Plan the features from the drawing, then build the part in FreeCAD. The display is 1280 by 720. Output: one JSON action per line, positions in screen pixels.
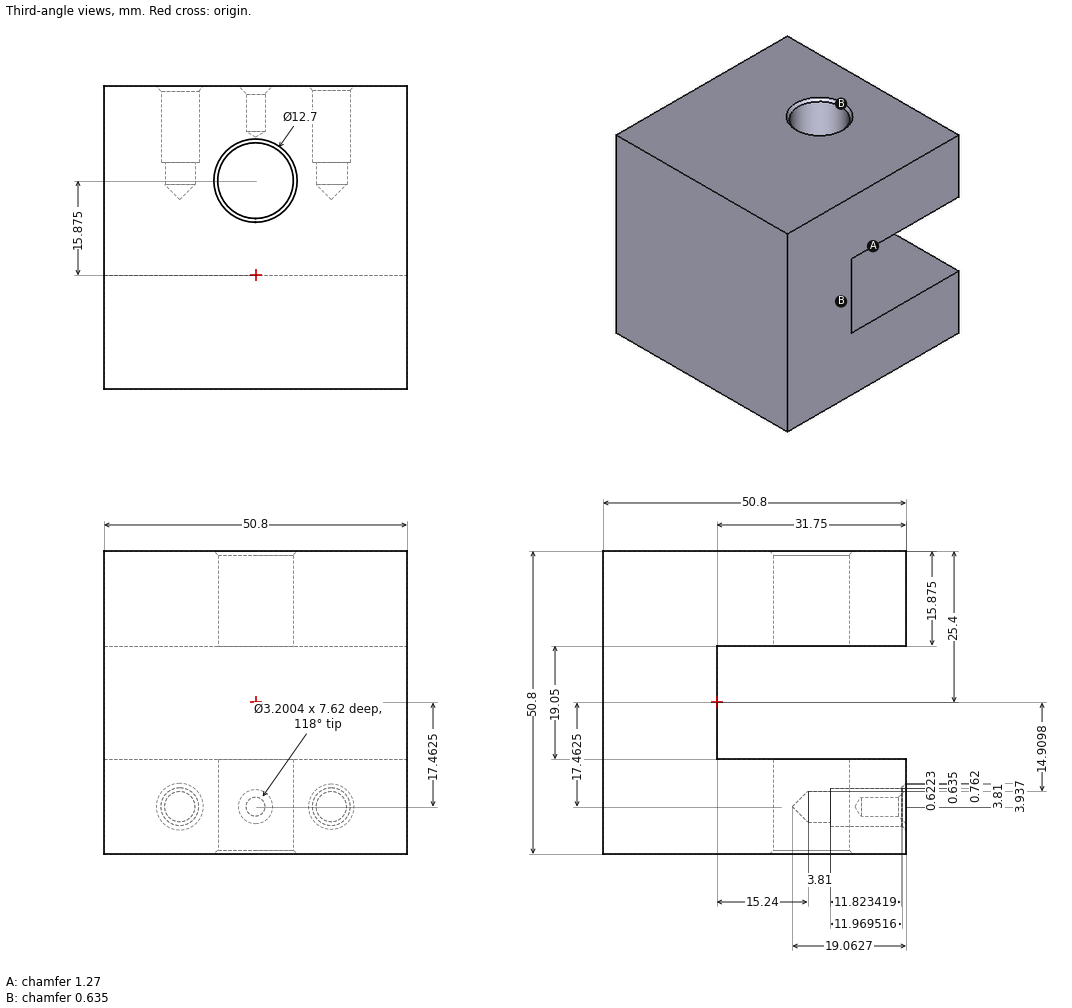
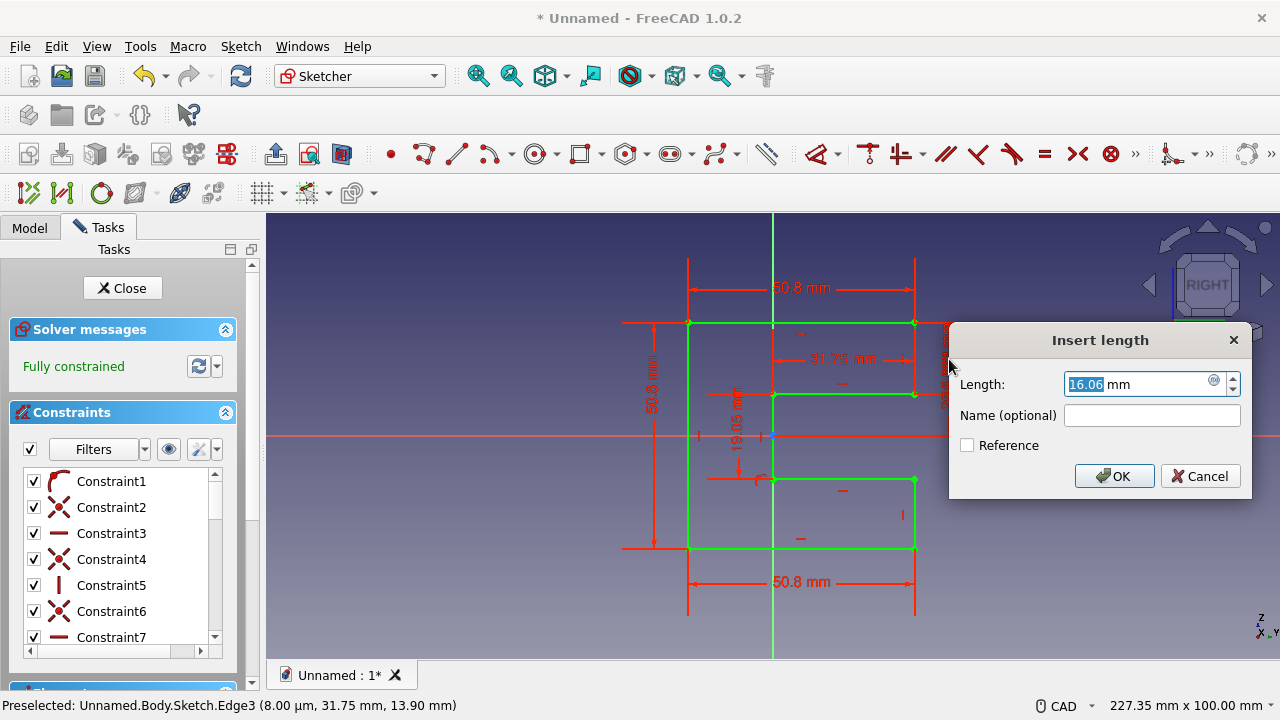
{"action": "type", "text": "15.875"}
{"action": "key", "text": "Return"}
{"action": "key", "text": "Escape"}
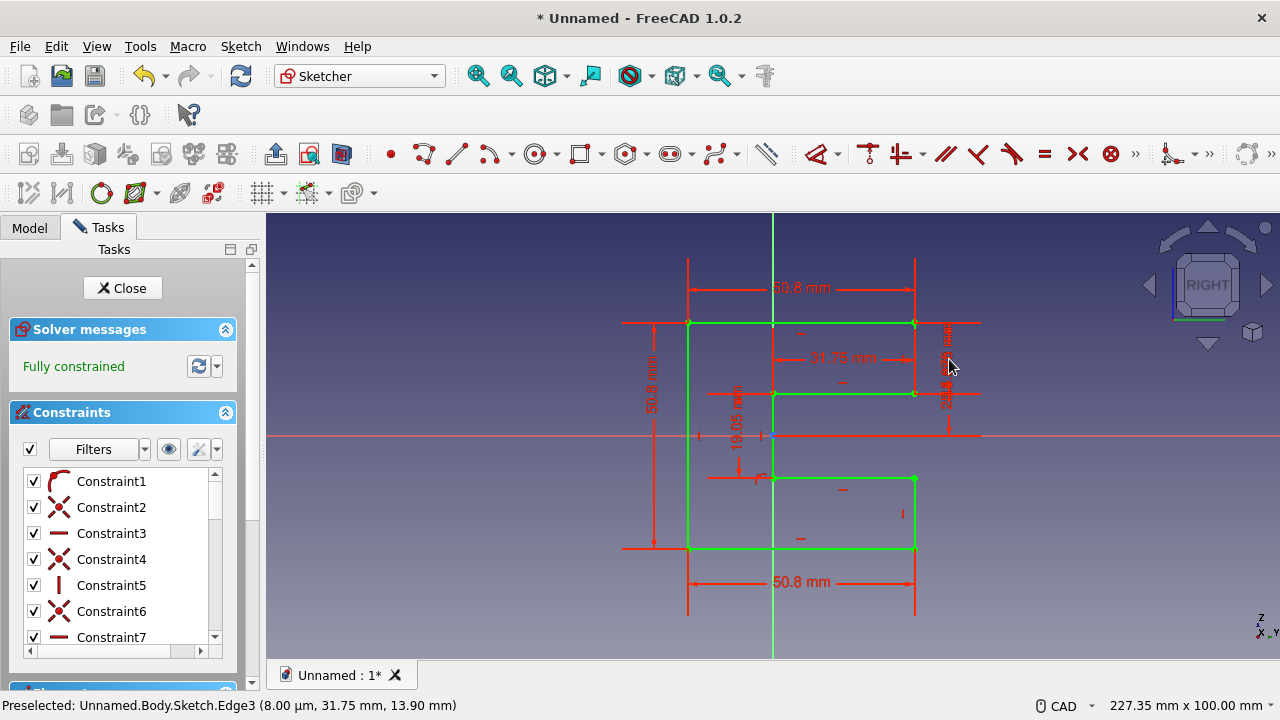
{"action": "left_click", "coordinate": [123, 288]}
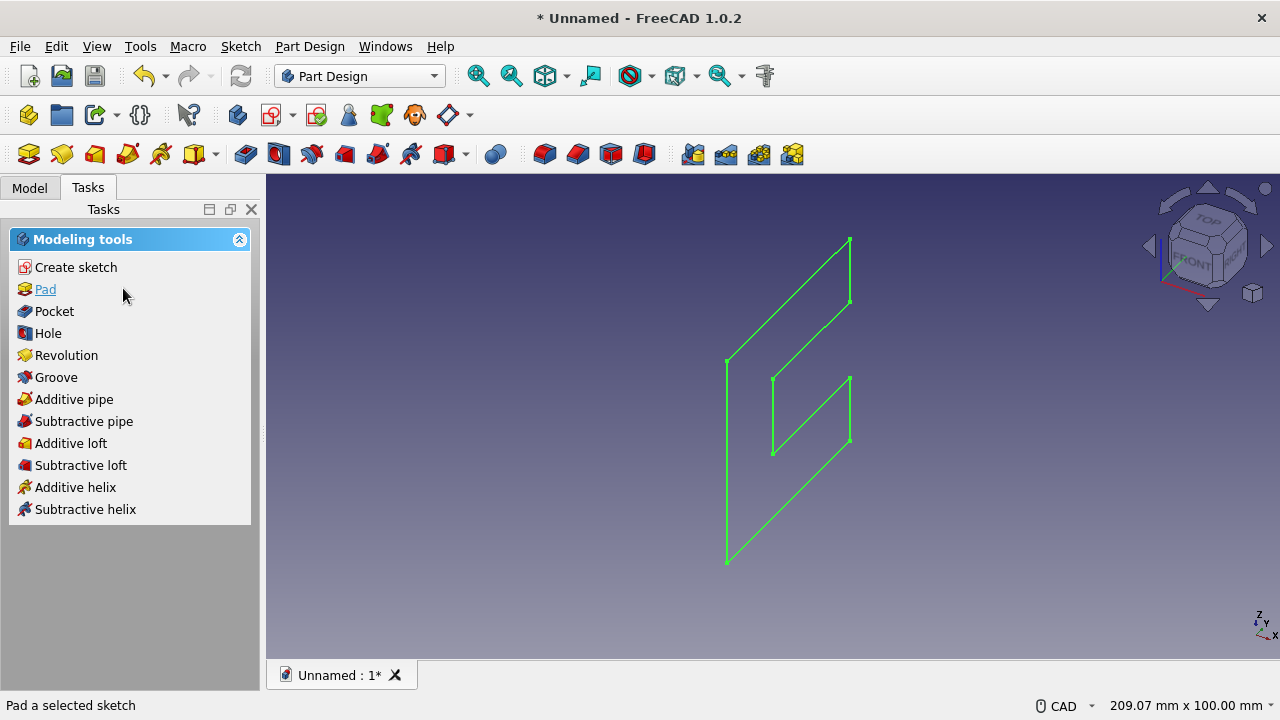
{"action": "left_click", "coordinate": [29, 154]}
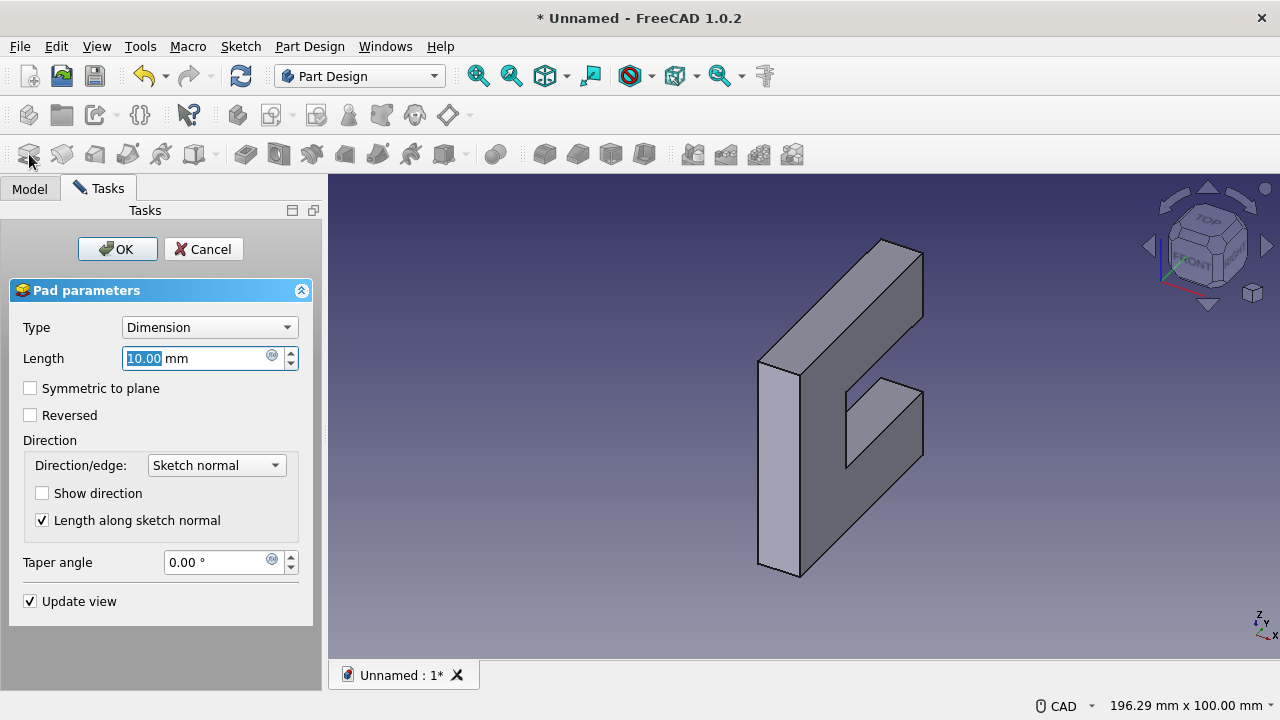
{"action": "type", "text": "50.8"}
{"action": "key", "text": "Tab"}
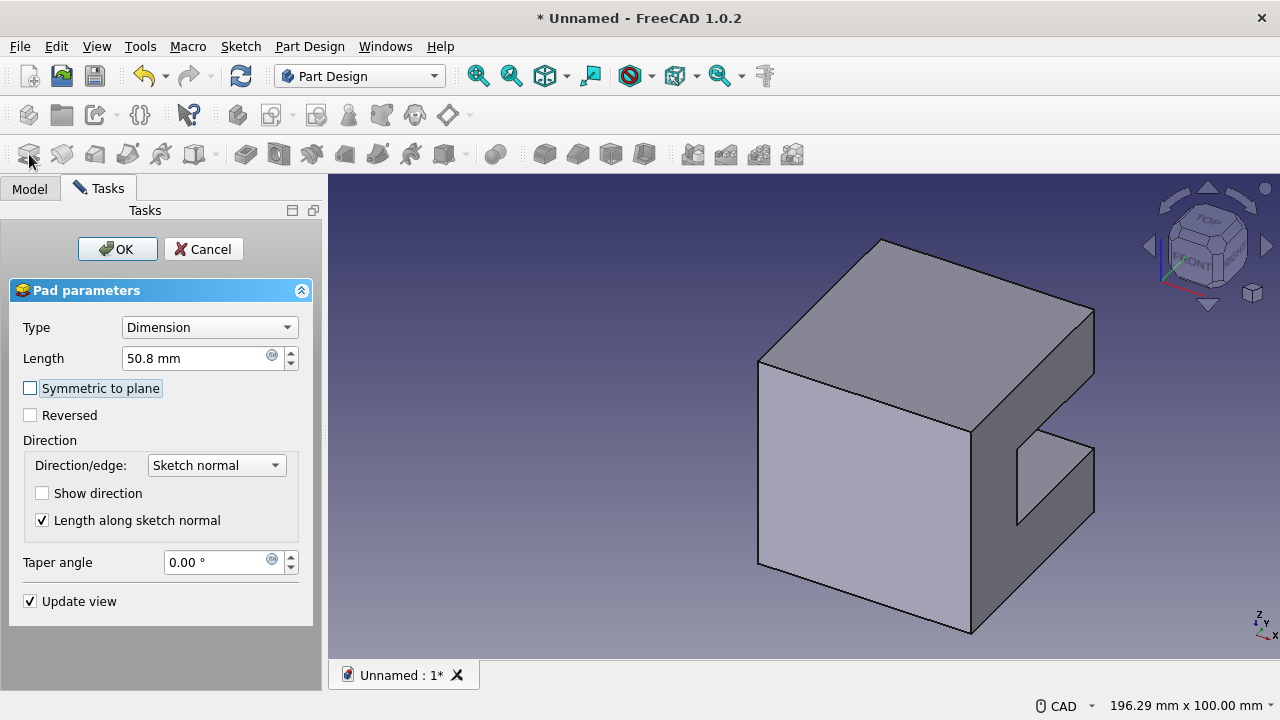
{"action": "left_click", "coordinate": [31, 388]}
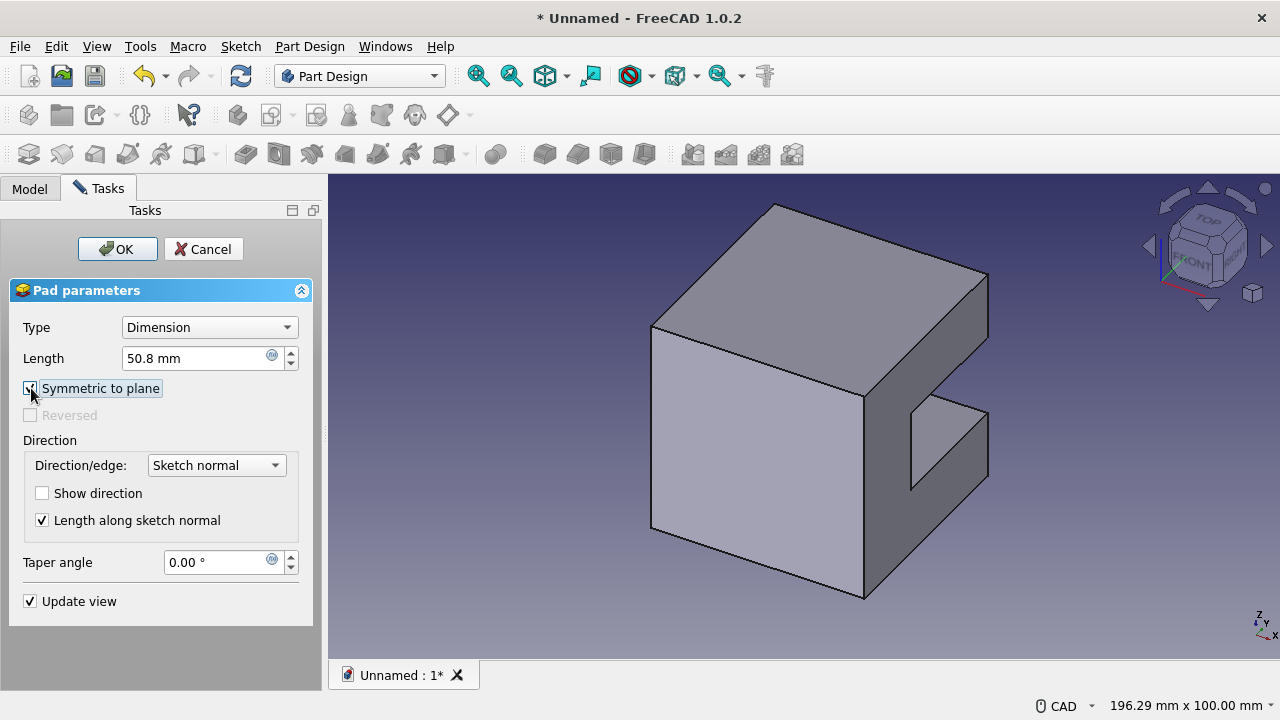
{"action": "left_click", "coordinate": [118, 249]}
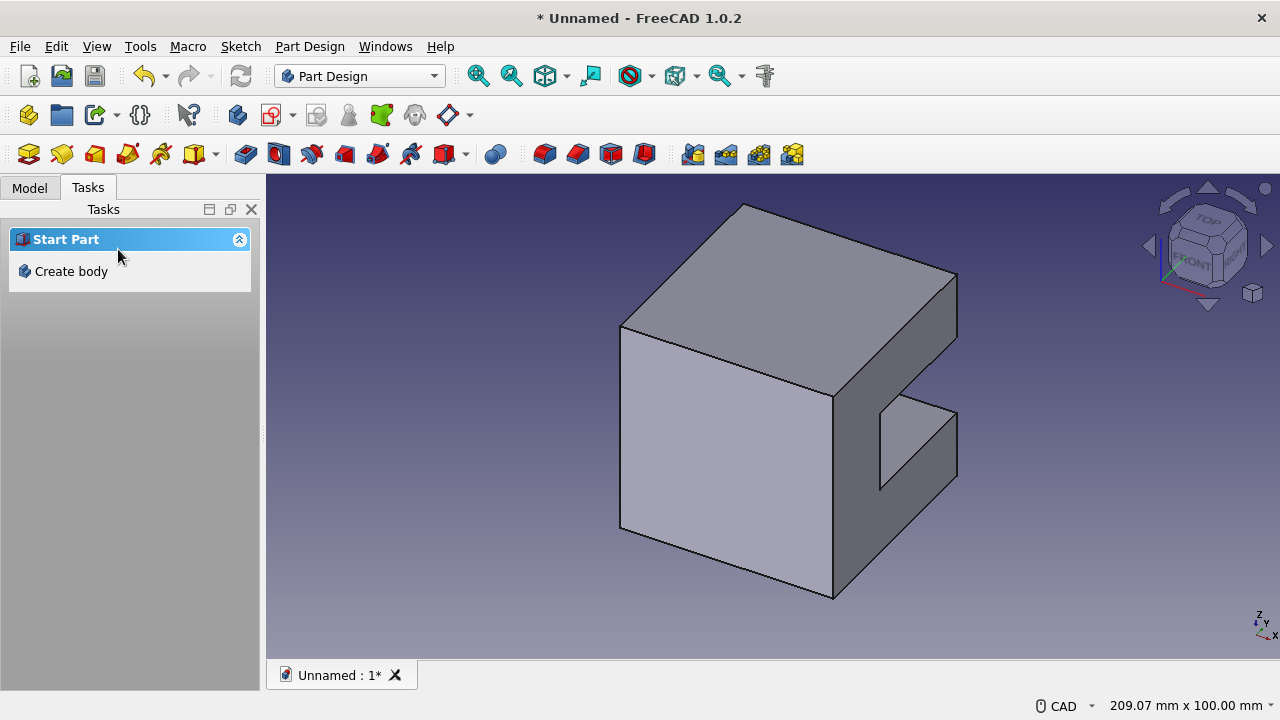
{"action": "key", "text": "4"}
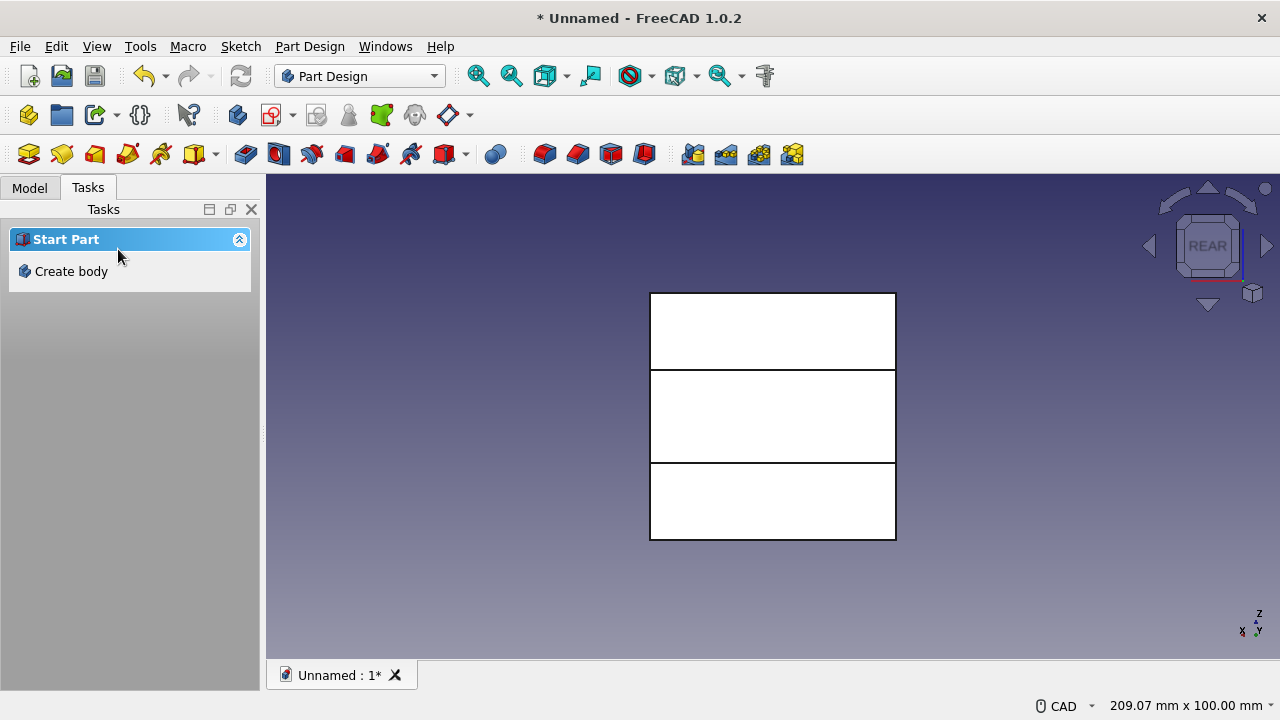
{"action": "left_click", "coordinate": [808, 331]}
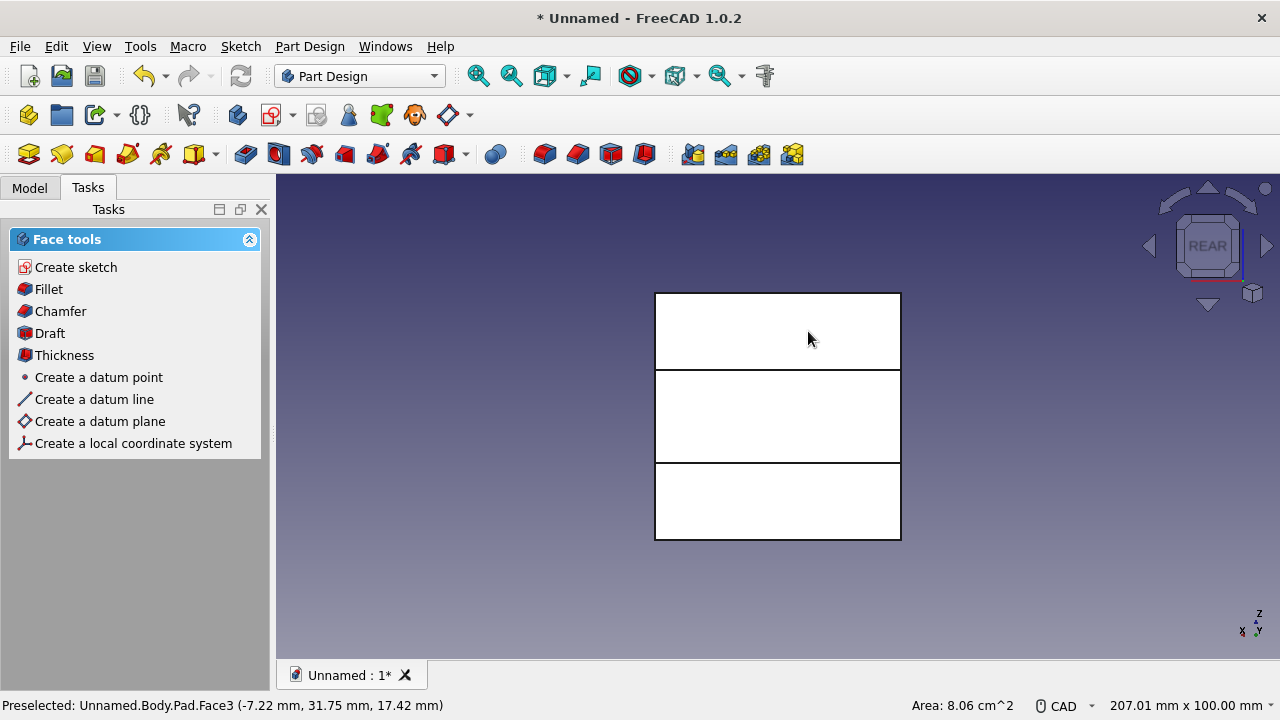
{"action": "left_click", "coordinate": [270, 116]}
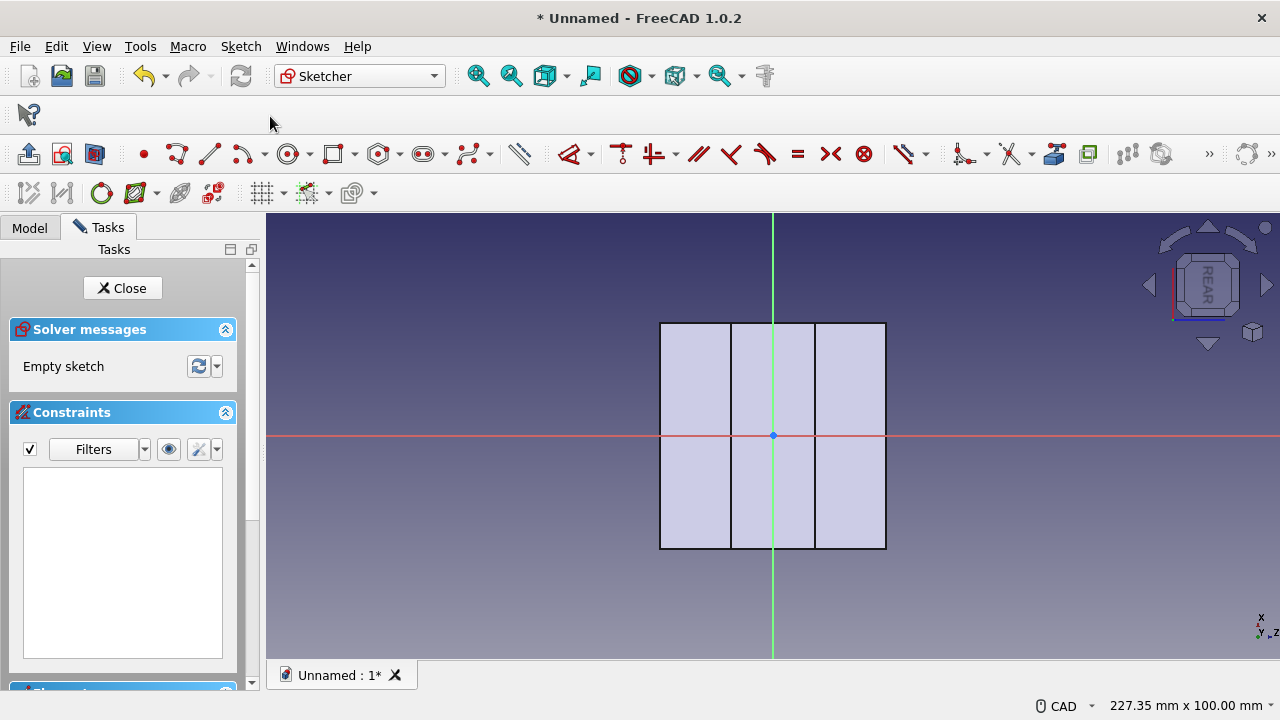
{"action": "scroll", "coordinate": [695, 436], "scroll_direction": "up", "scroll_amount": 15}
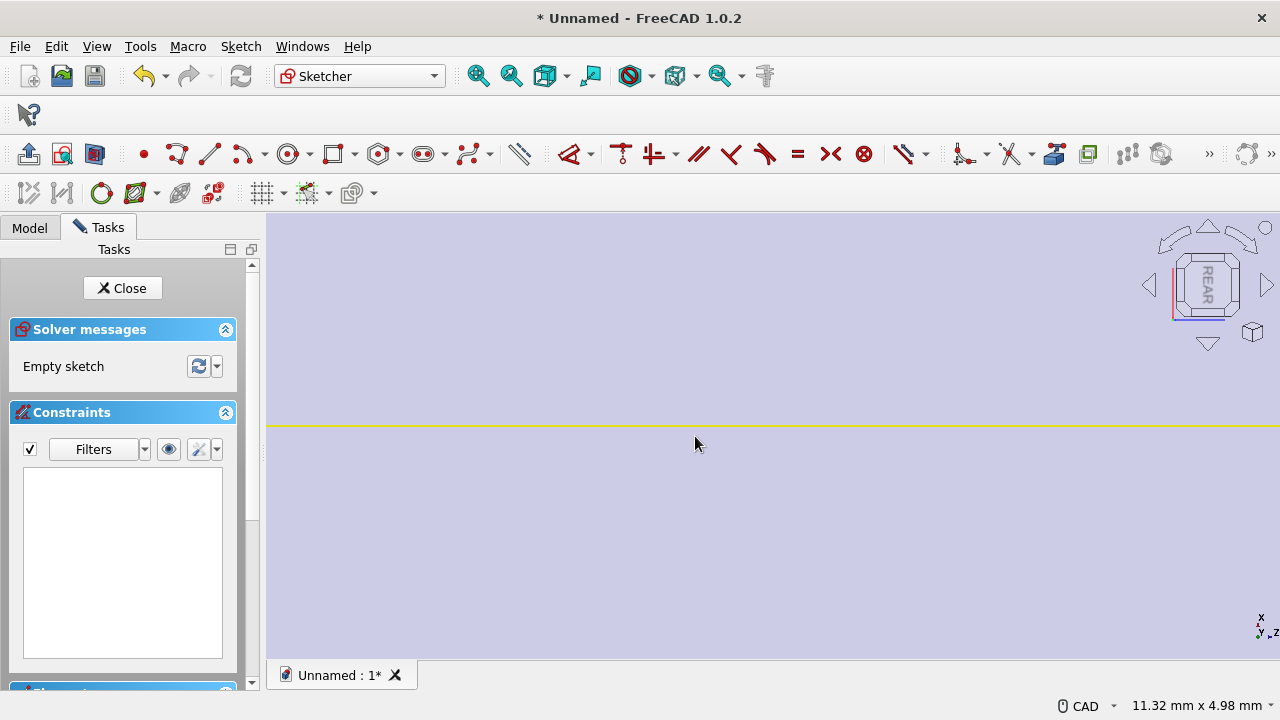
{"action": "left_click", "coordinate": [288, 154]}